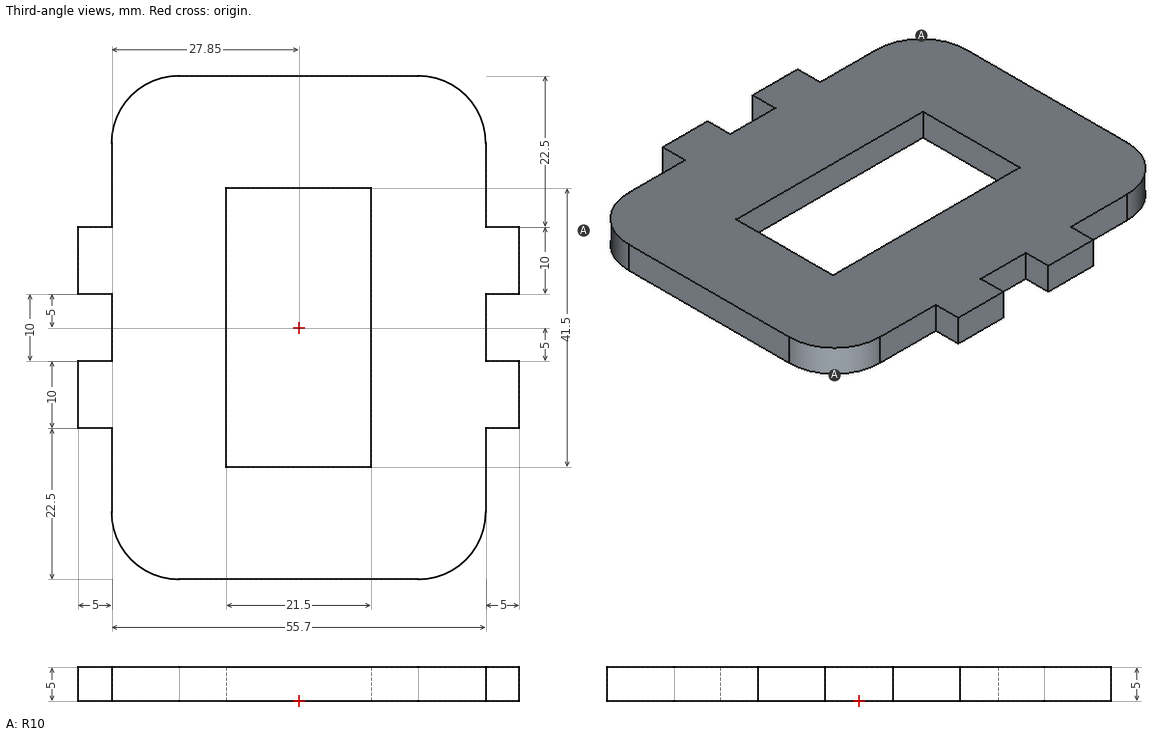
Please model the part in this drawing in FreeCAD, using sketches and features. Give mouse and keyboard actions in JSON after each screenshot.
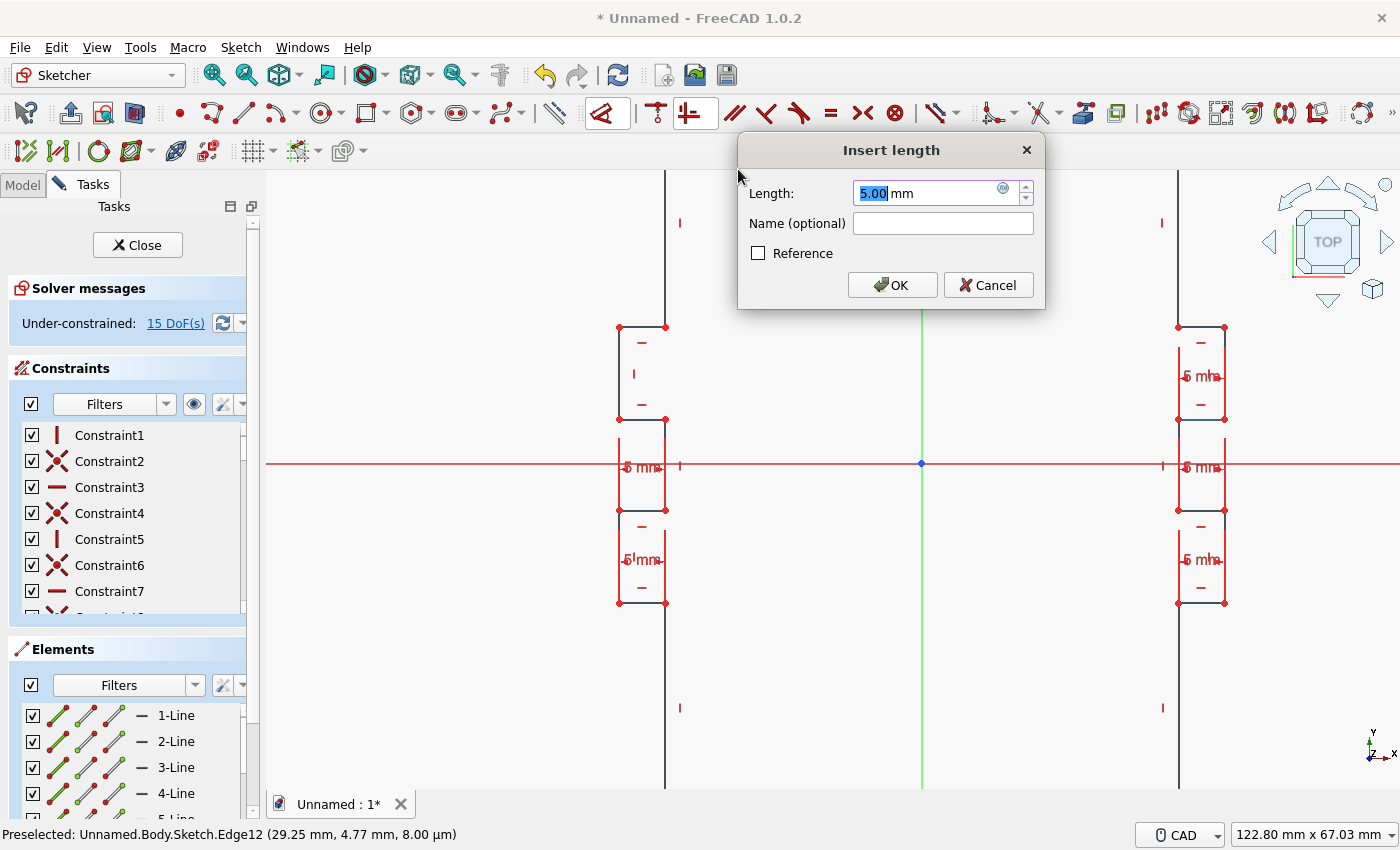
{"action": "type", "text": "5"}
{"action": "key", "text": "Return"}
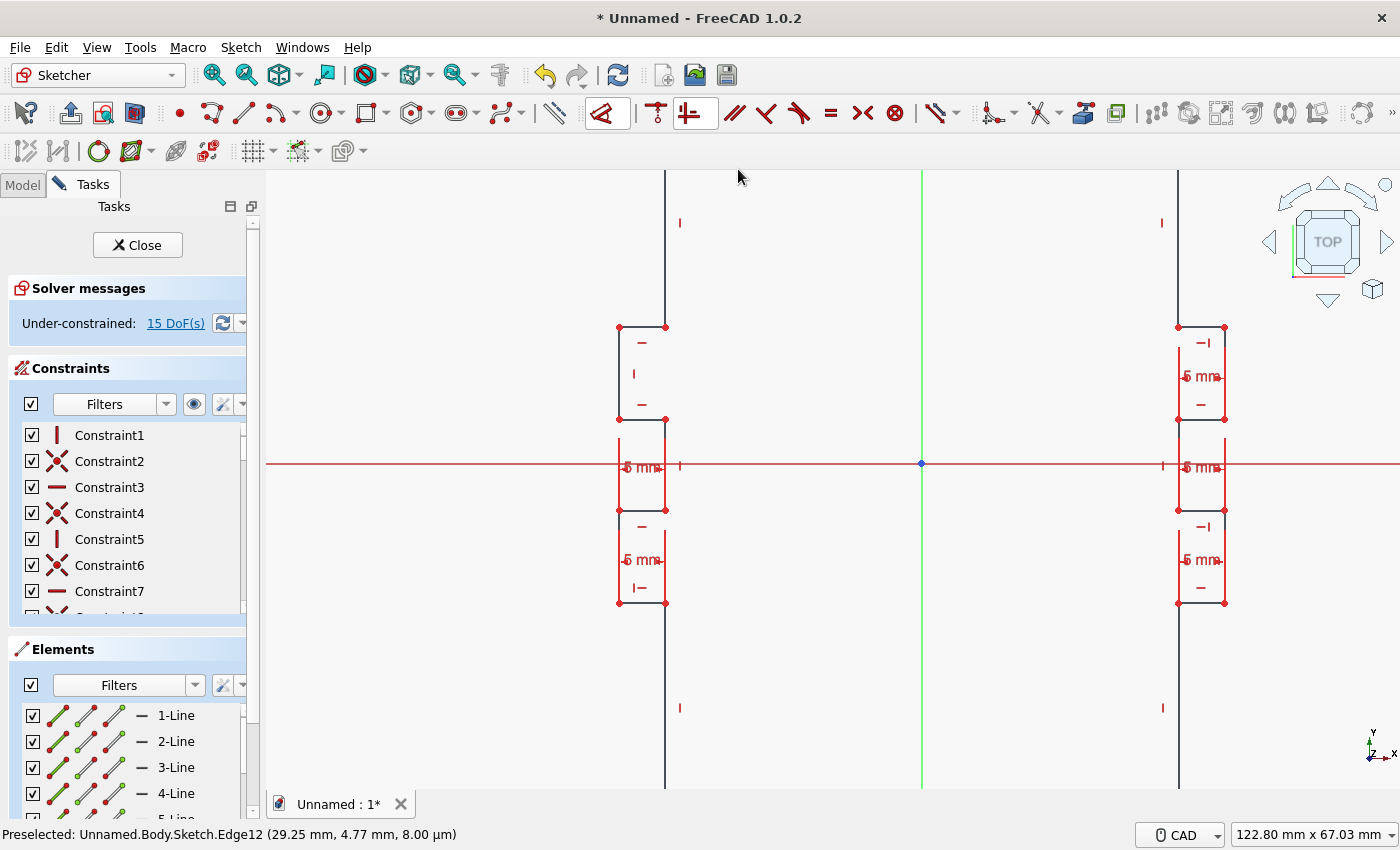
{"action": "left_click", "coordinate": [1211, 327]}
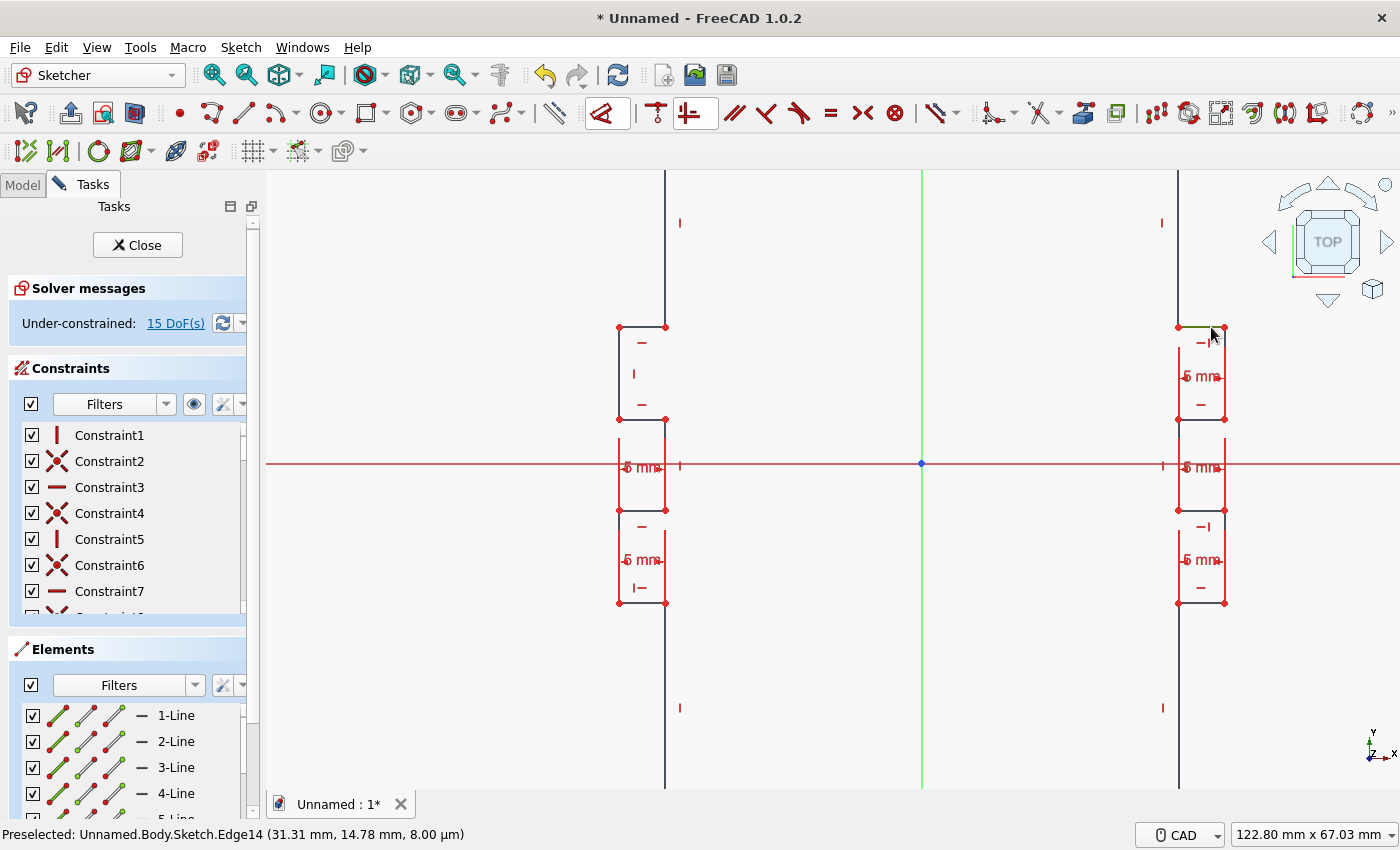
{"action": "key", "text": "l"}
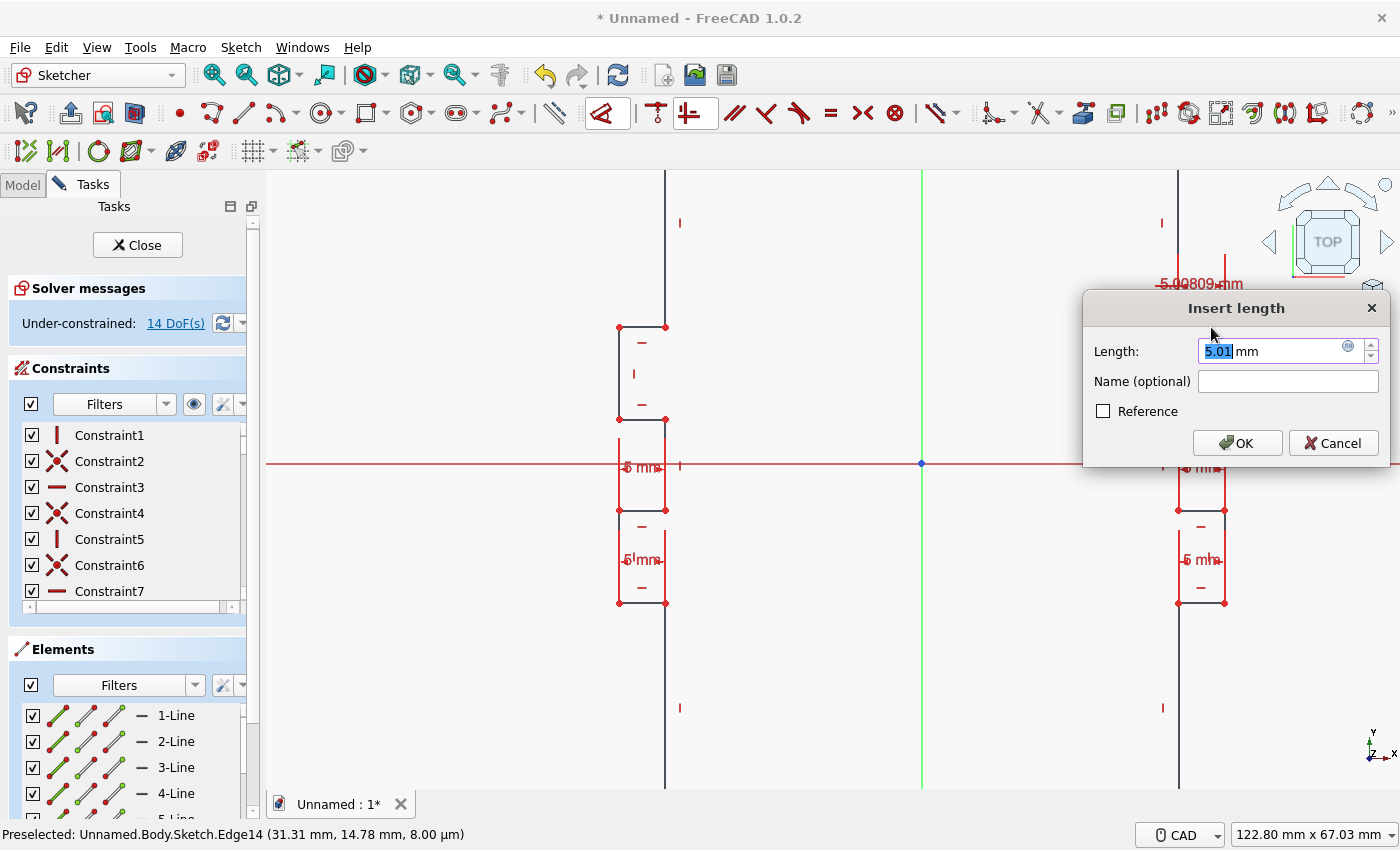
{"action": "type", "text": "5"}
{"action": "key", "text": "Return"}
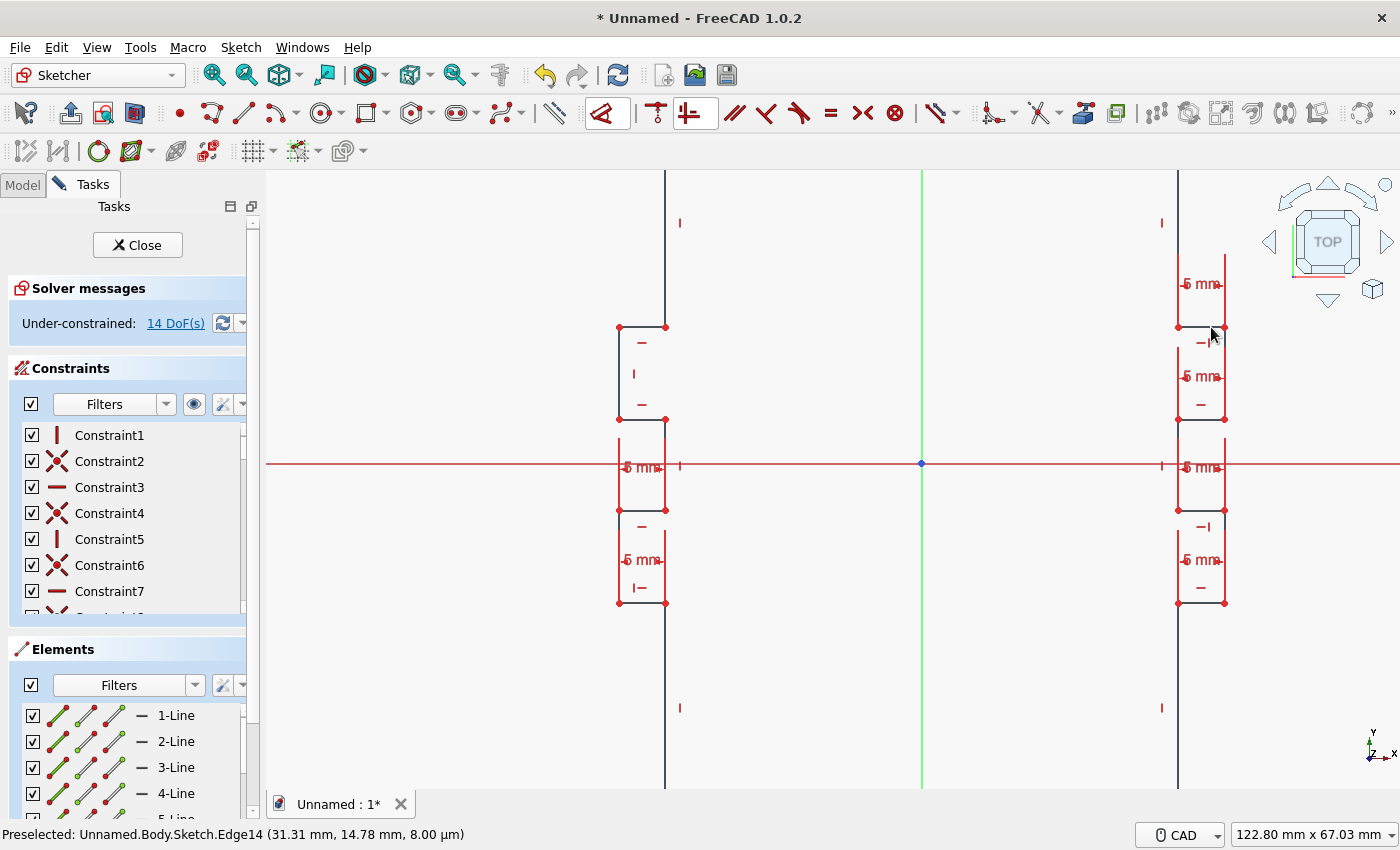
{"action": "left_click", "coordinate": [651, 327]}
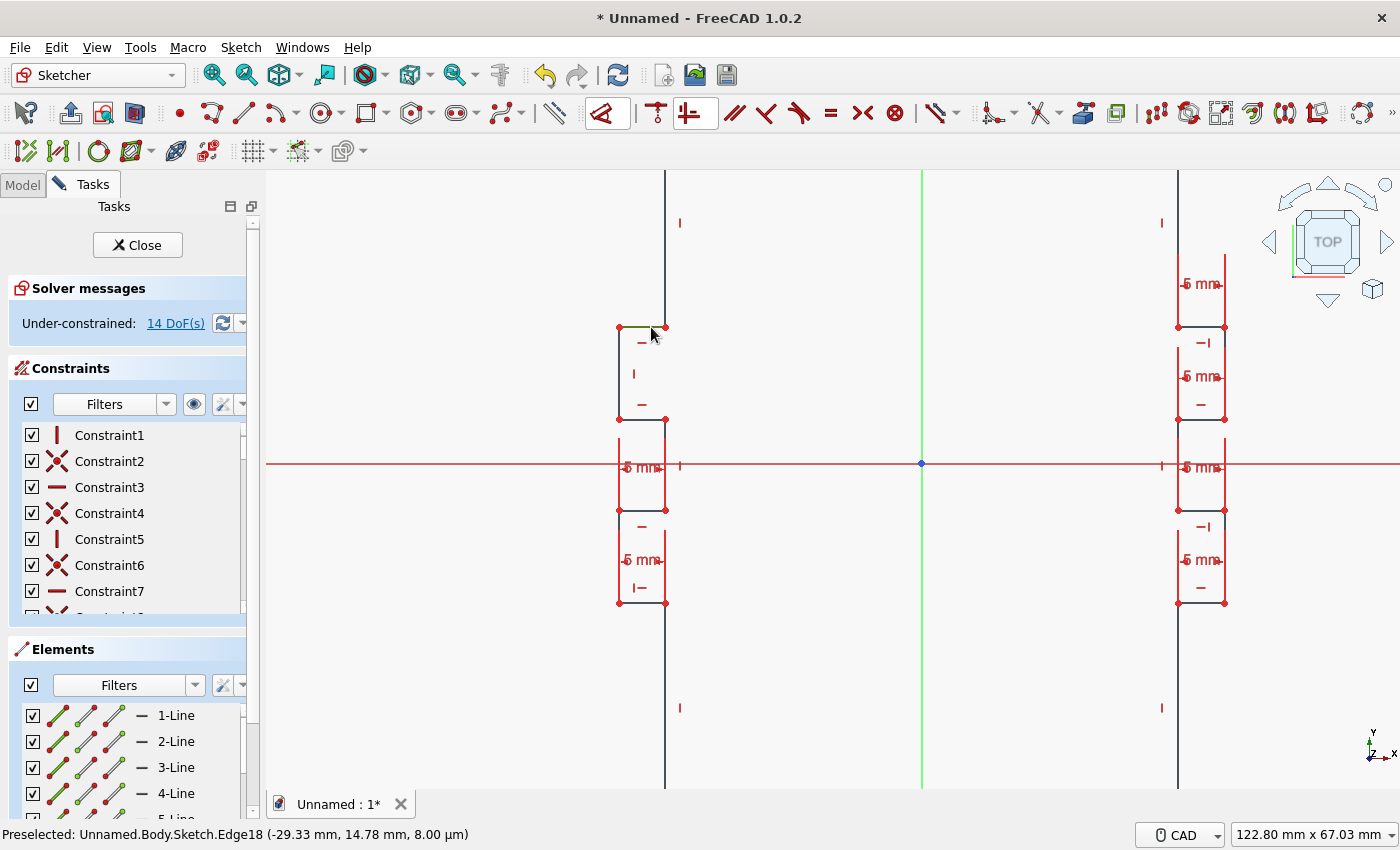
{"action": "left_click", "coordinate": [624, 114]}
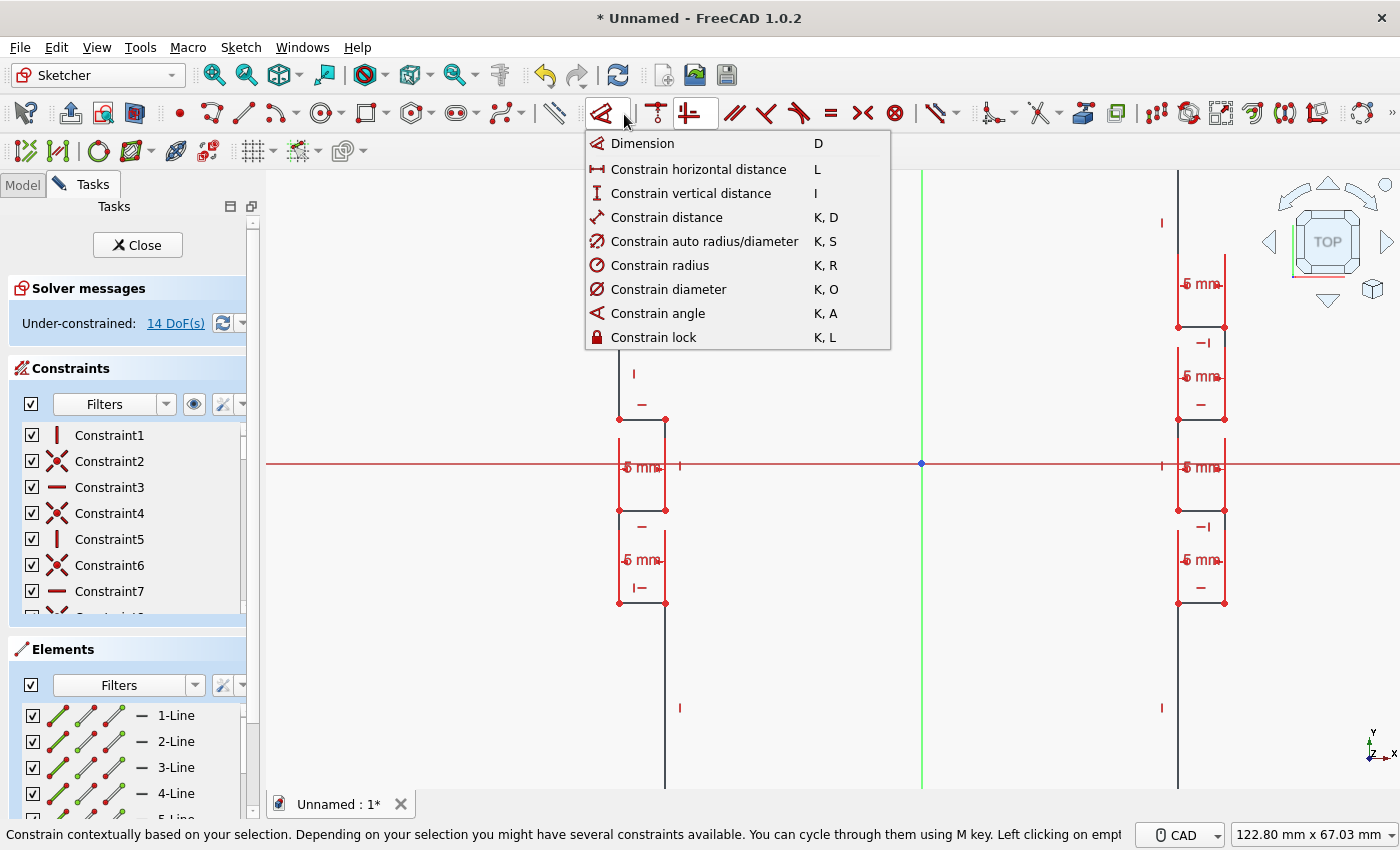
{"action": "left_click", "coordinate": [738, 169]}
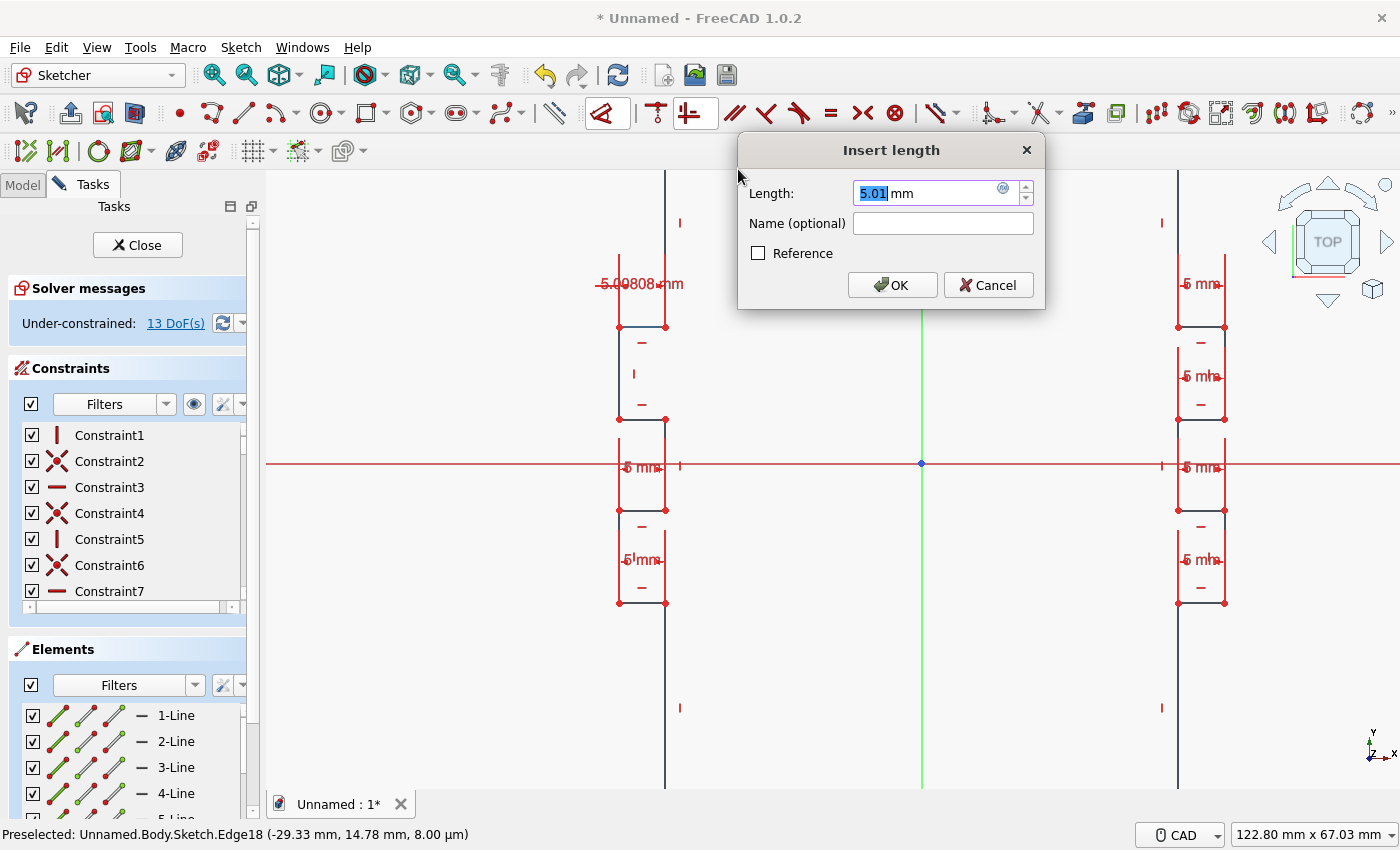
{"action": "type", "text": "5"}
{"action": "key", "text": "Return"}